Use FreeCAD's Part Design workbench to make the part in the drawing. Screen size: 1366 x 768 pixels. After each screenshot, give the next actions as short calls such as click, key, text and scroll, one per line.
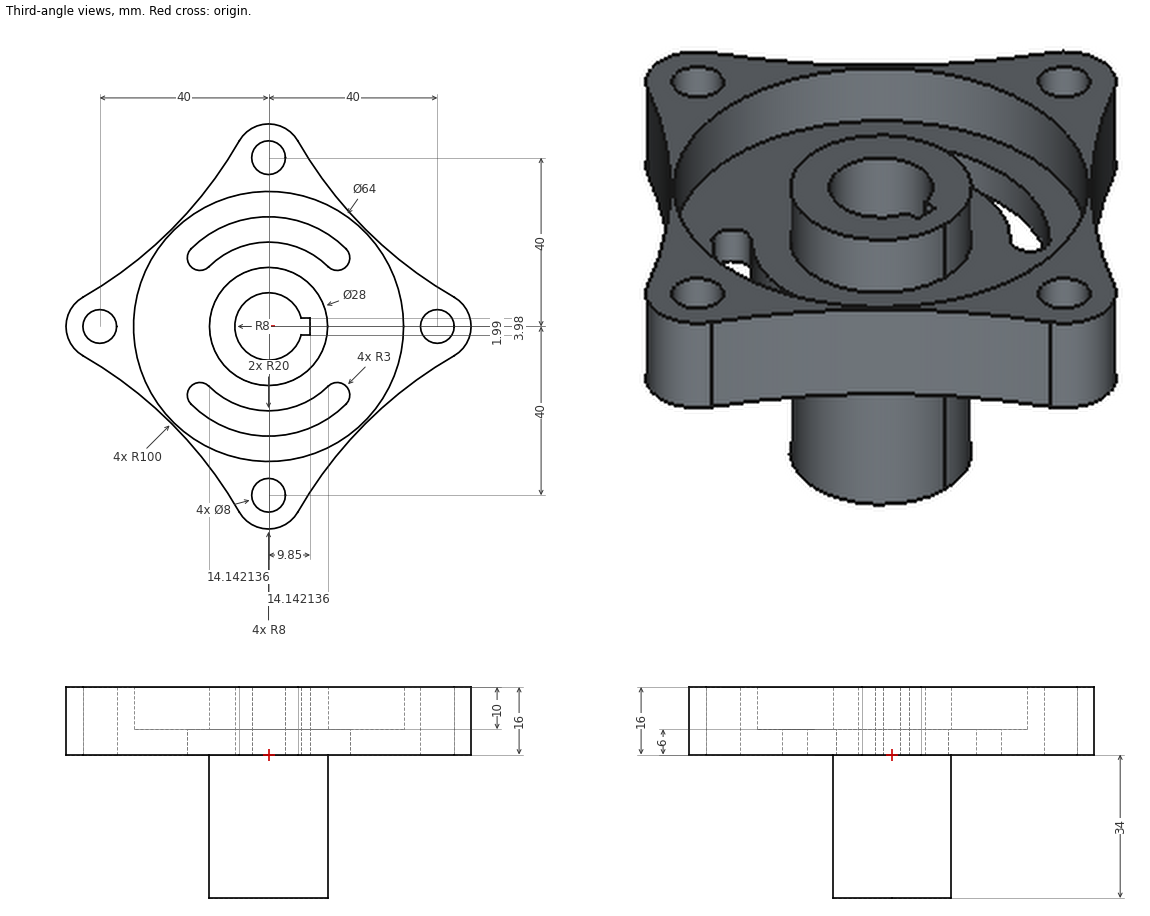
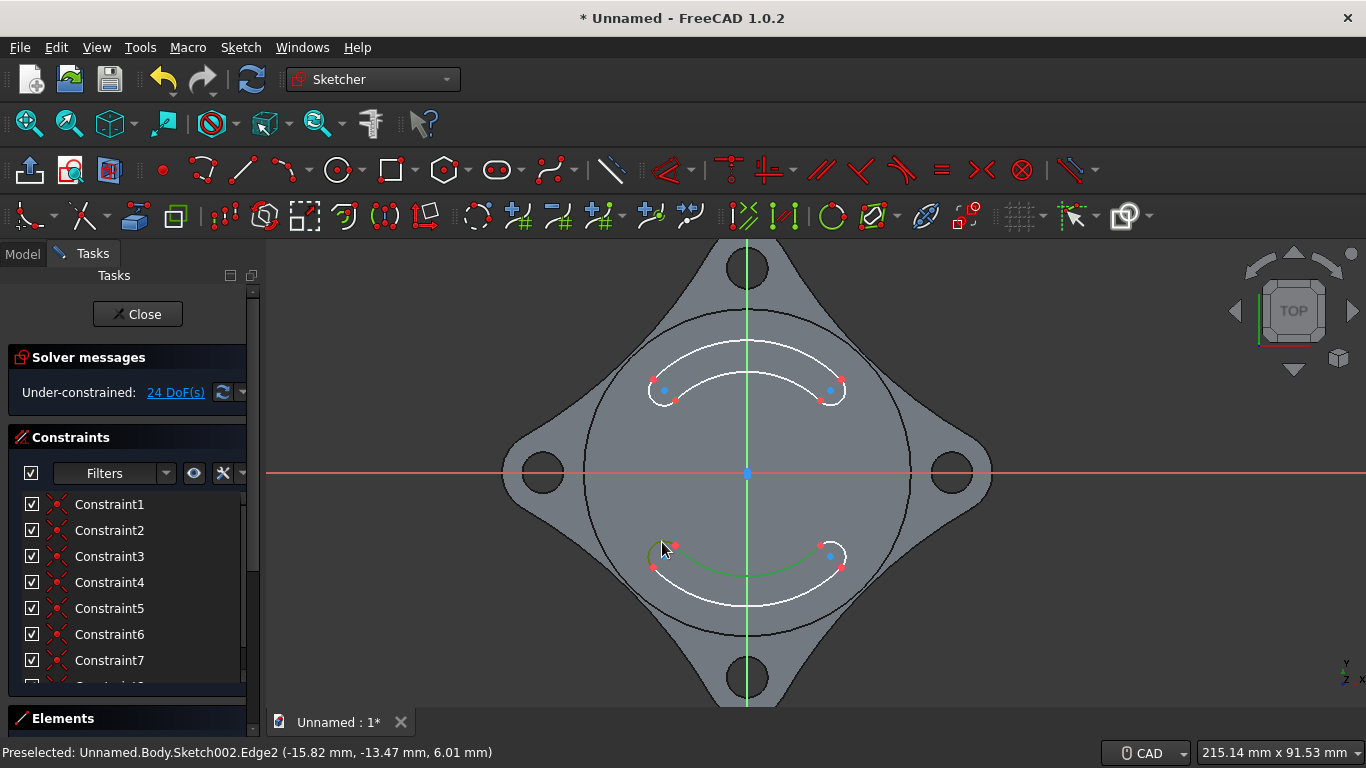
click(902, 170)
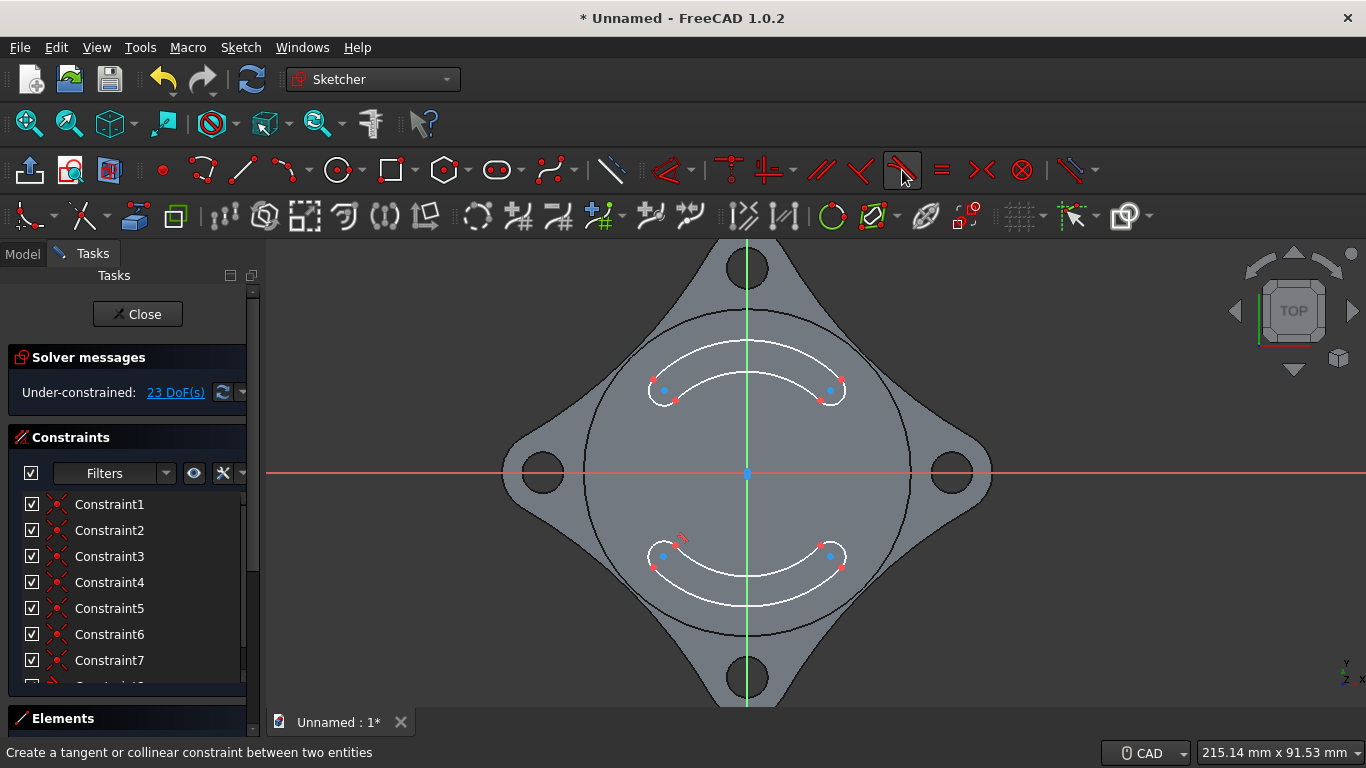
click(716, 571)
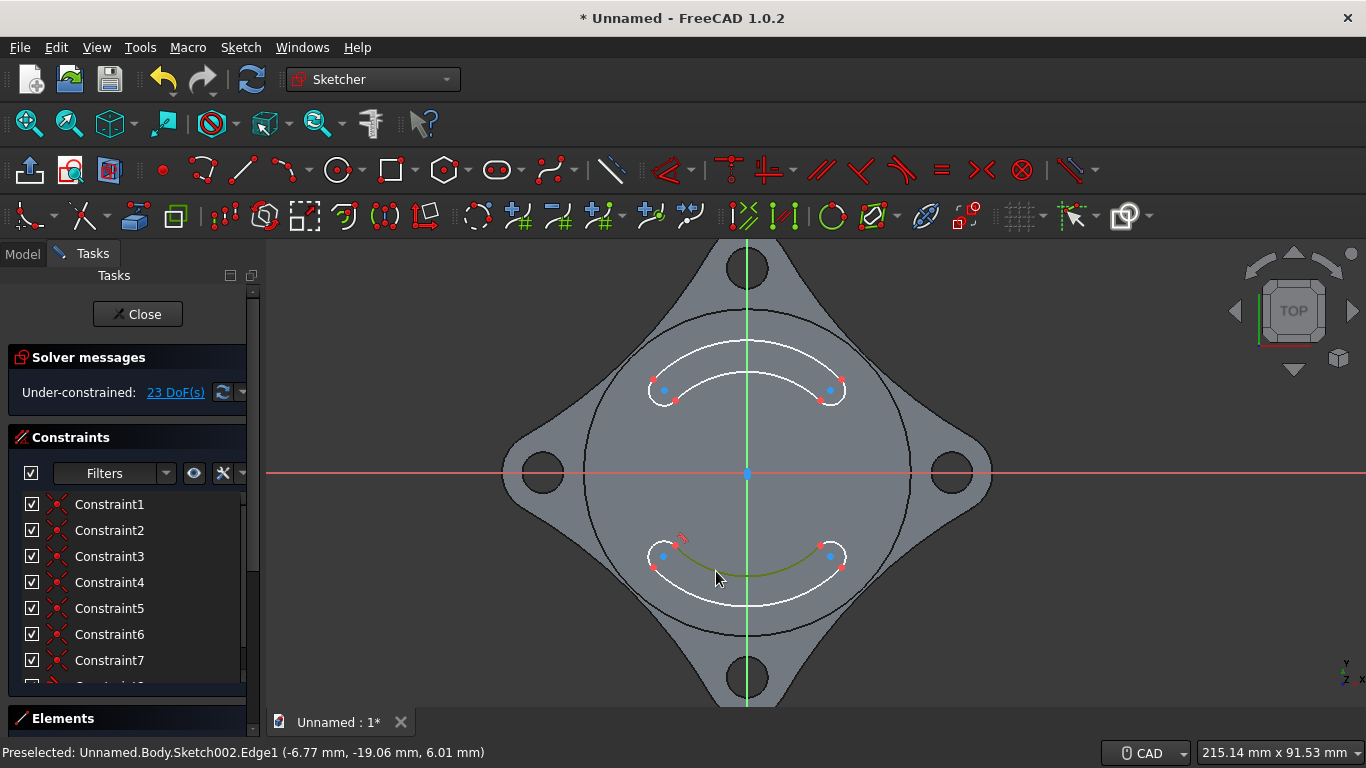
click(846, 555)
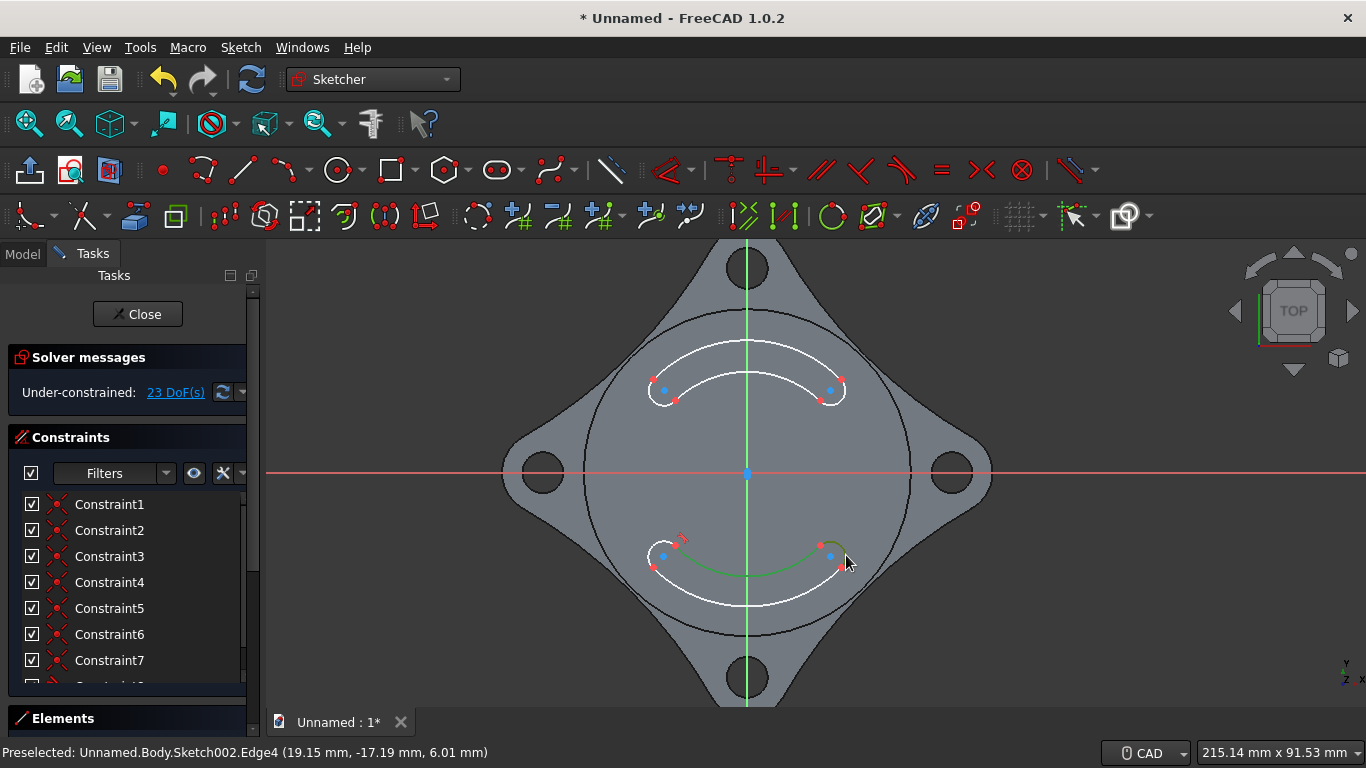
click(902, 170)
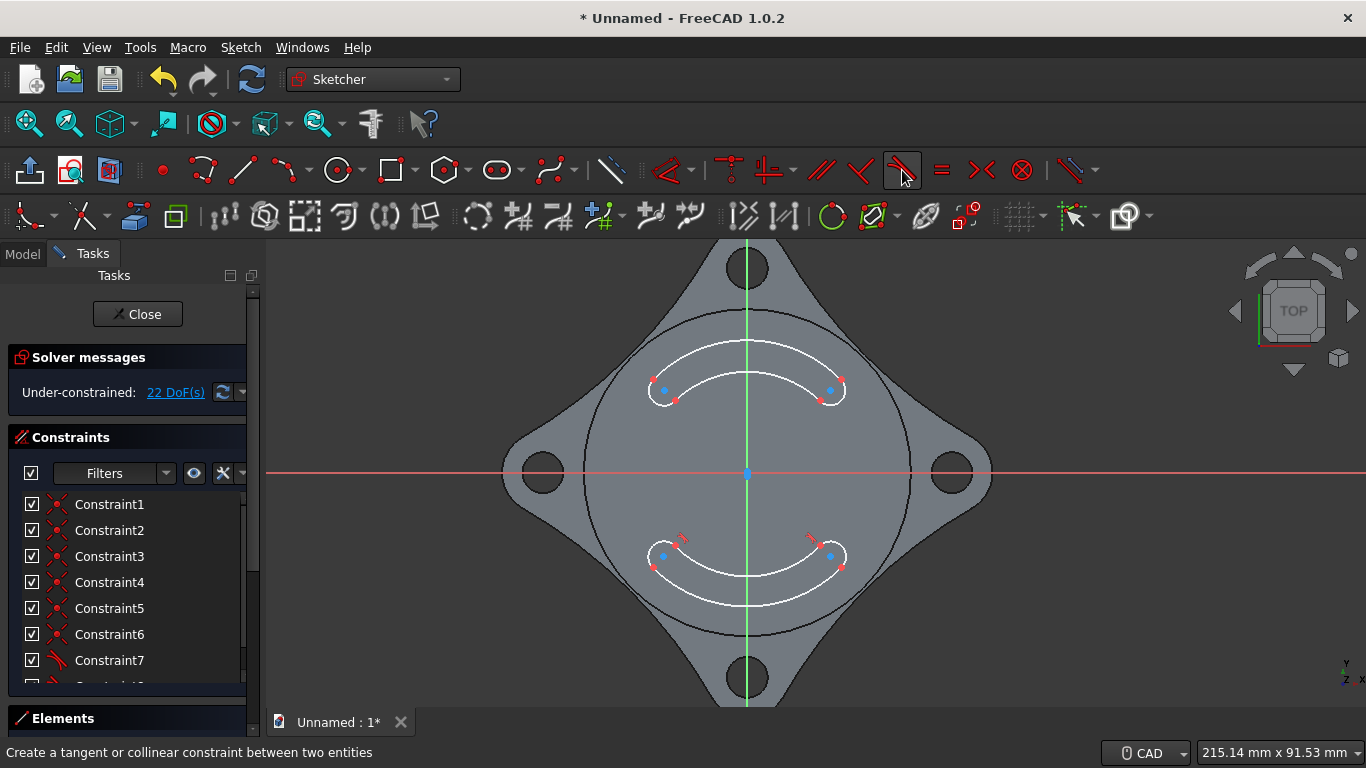
click(662, 542)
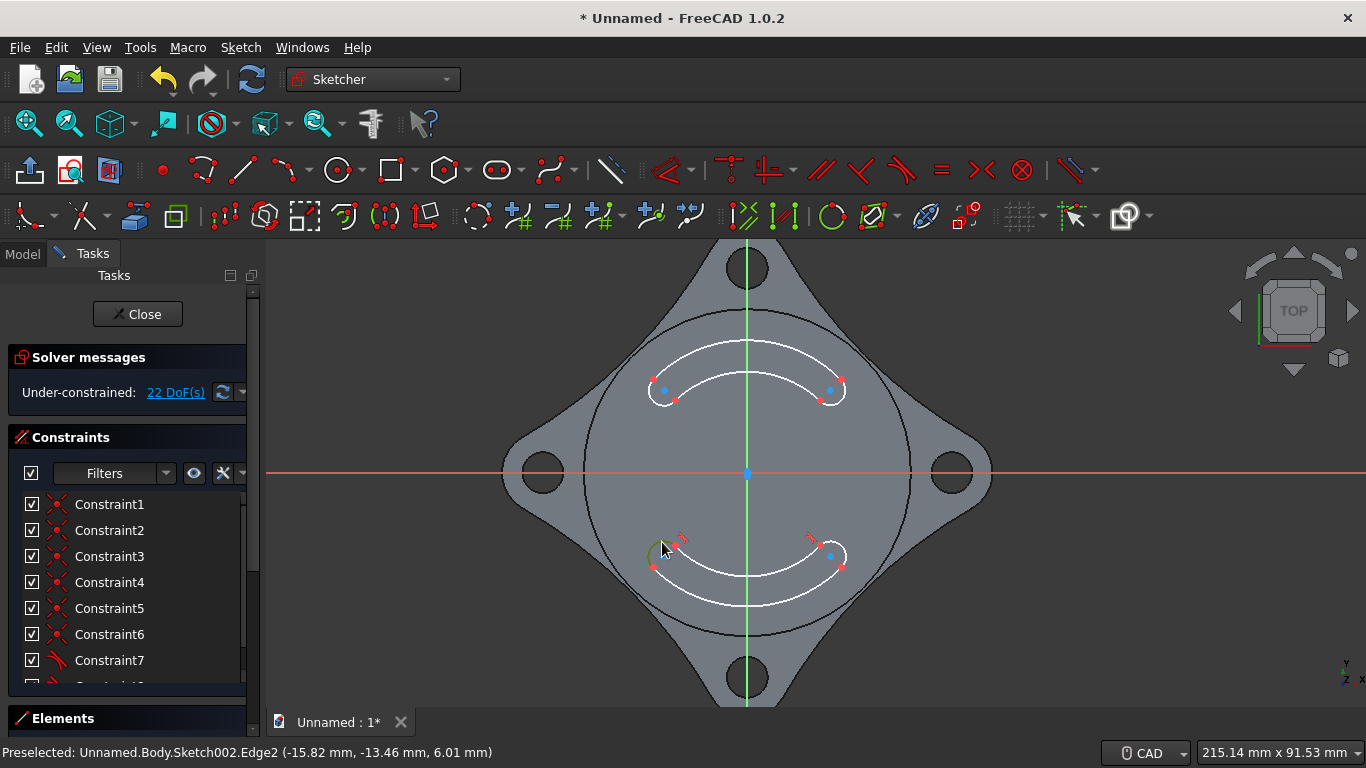
click(706, 600)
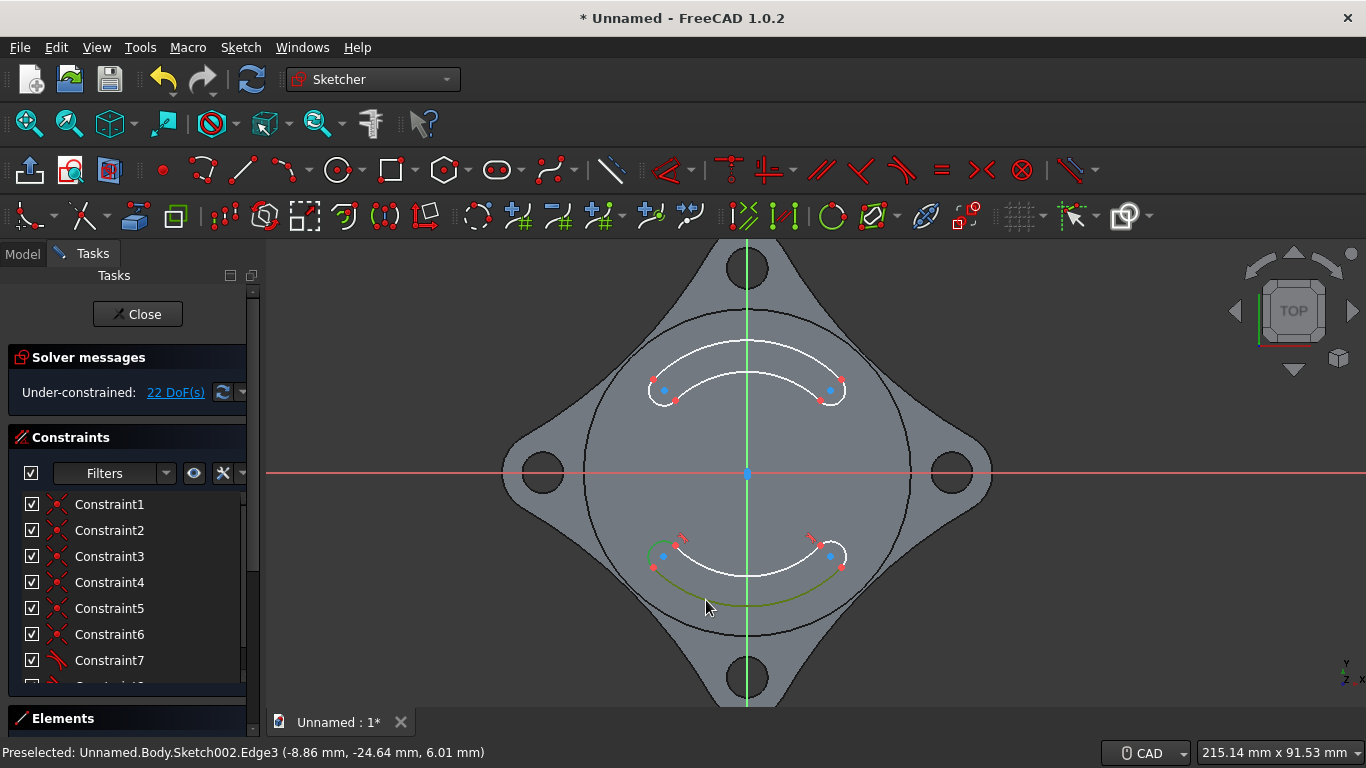
key(t)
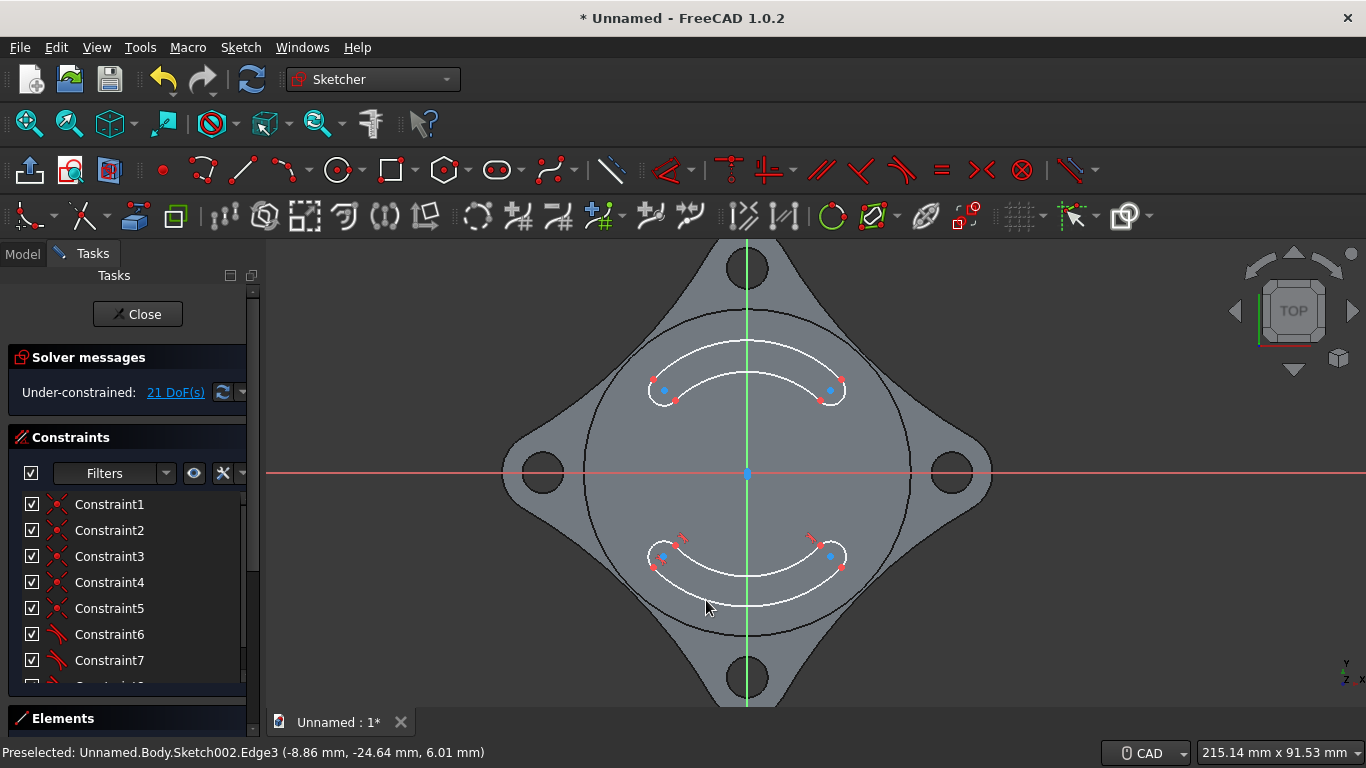
click(706, 600)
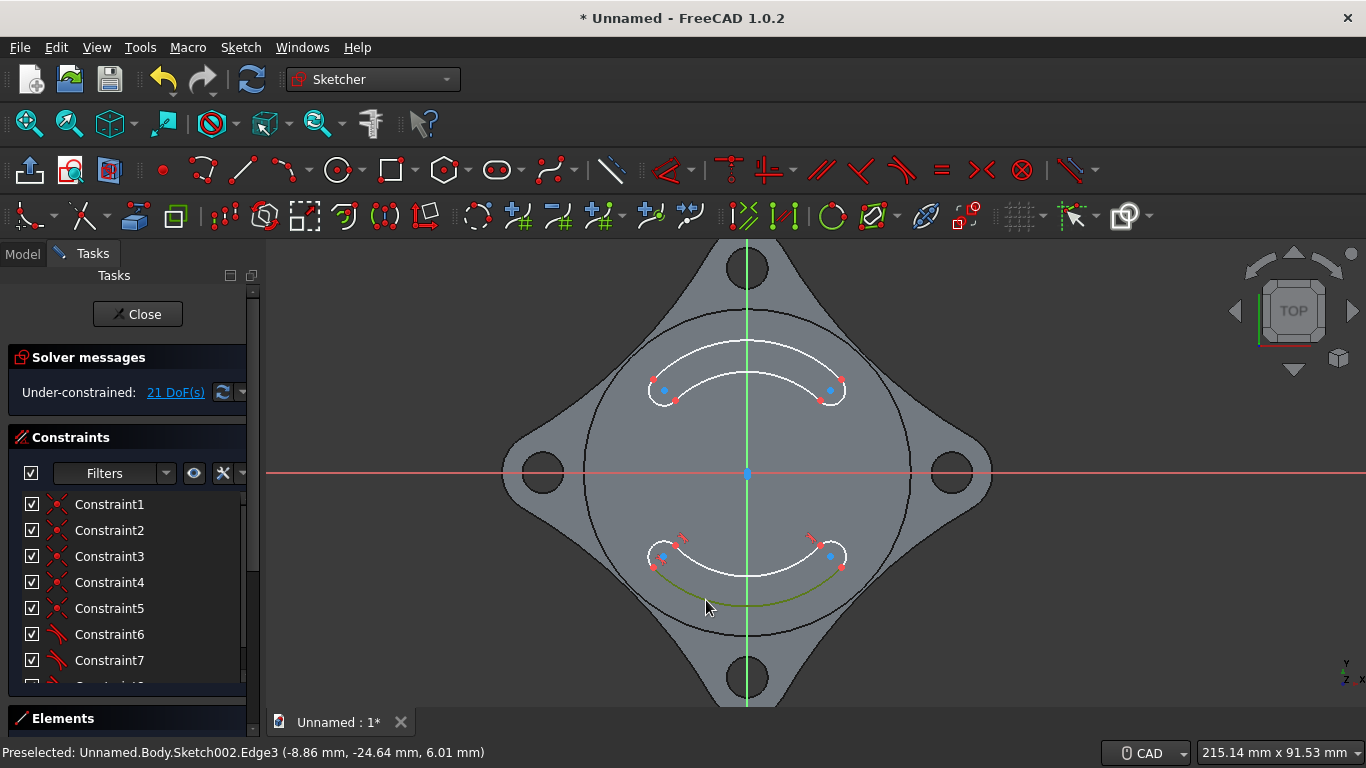
click(846, 555)